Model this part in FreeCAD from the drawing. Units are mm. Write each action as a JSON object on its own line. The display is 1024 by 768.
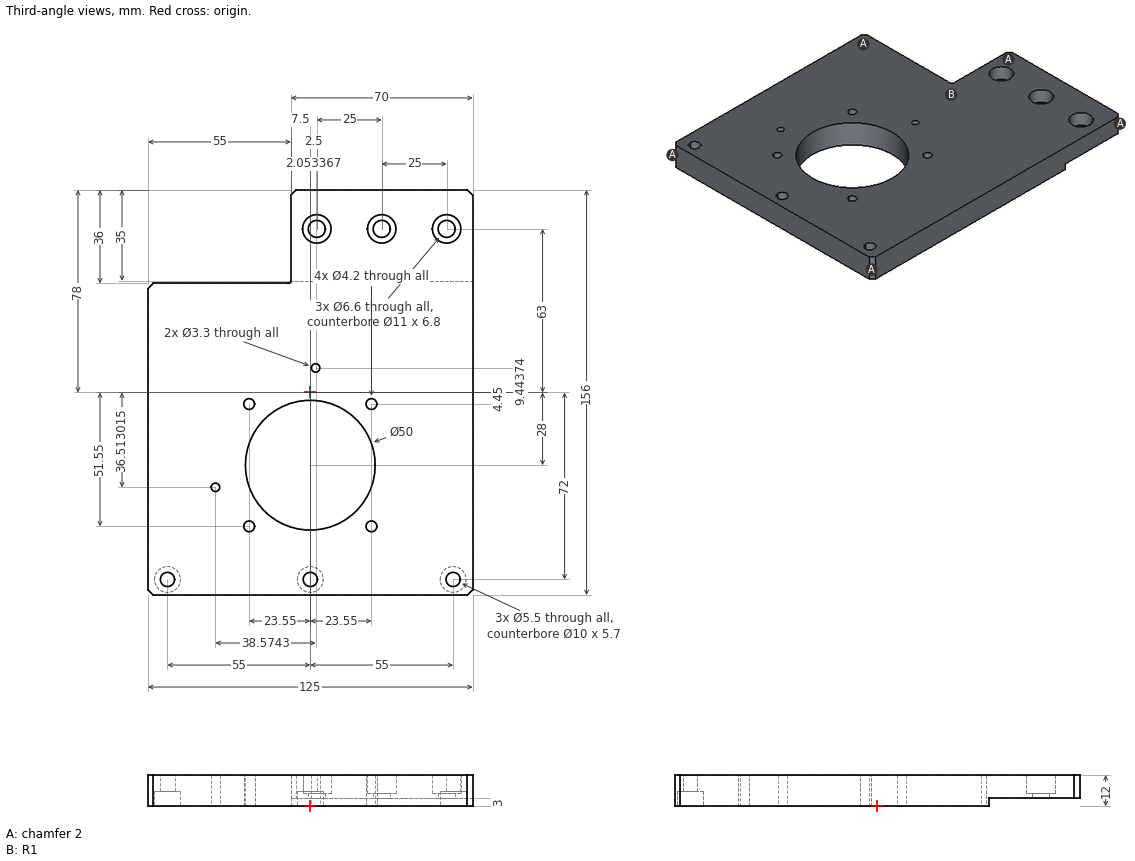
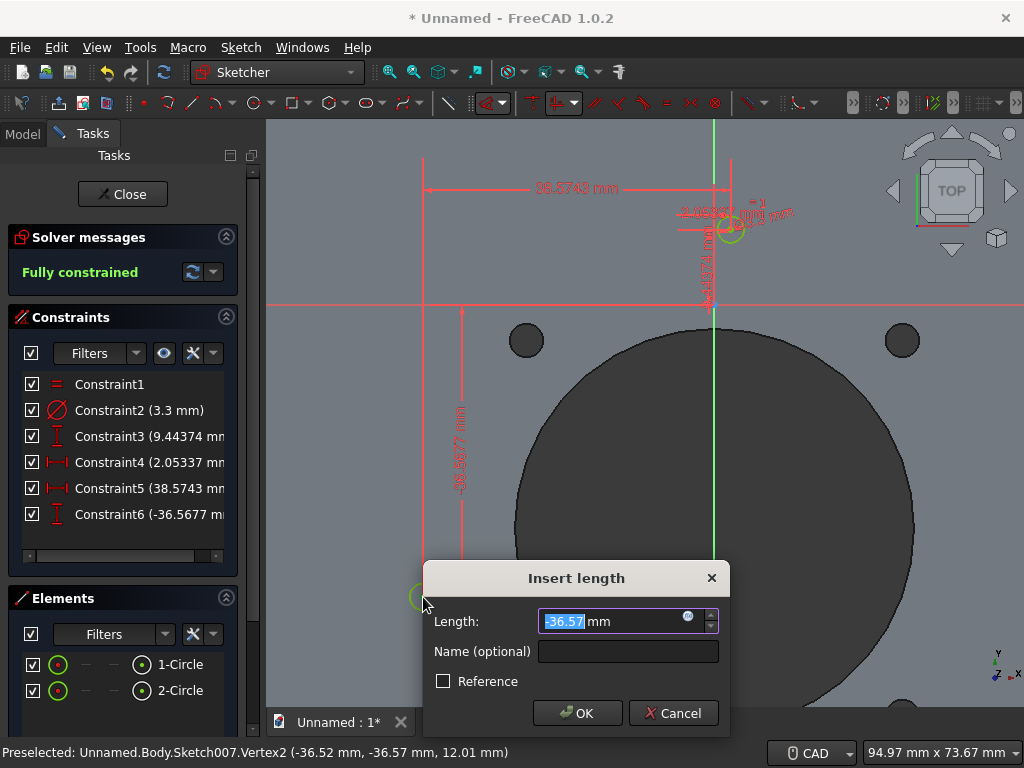
{"action": "type", "text": "-36.513015"}
{"action": "key", "text": "Return"}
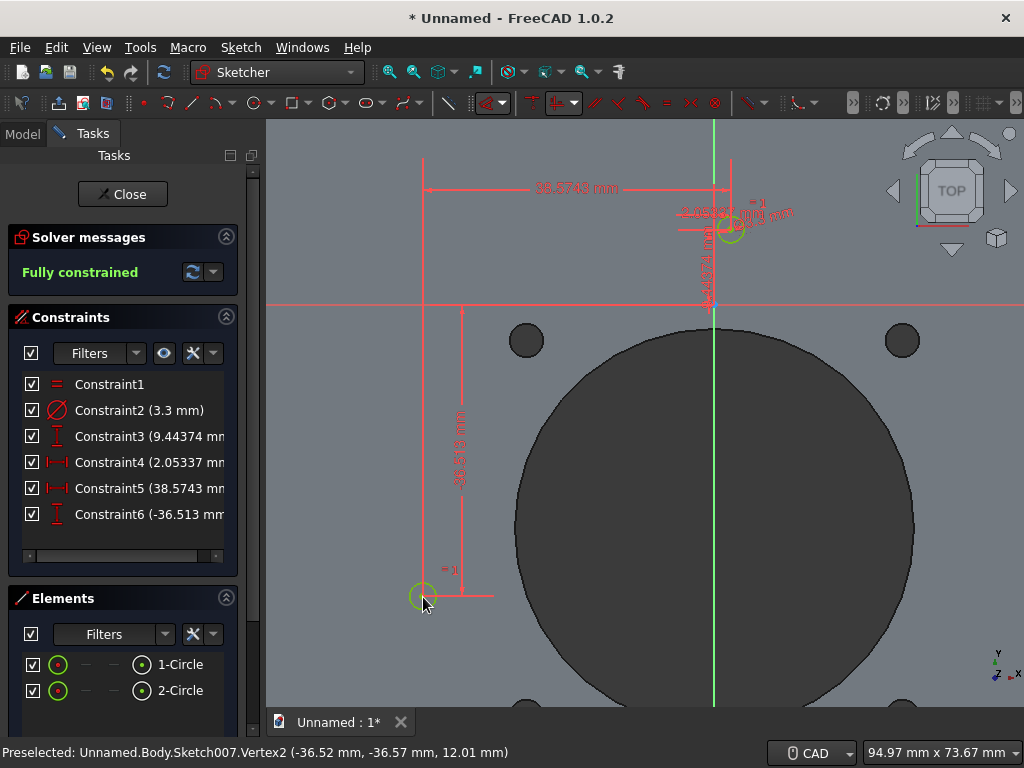
{"action": "left_click", "coordinate": [123, 194]}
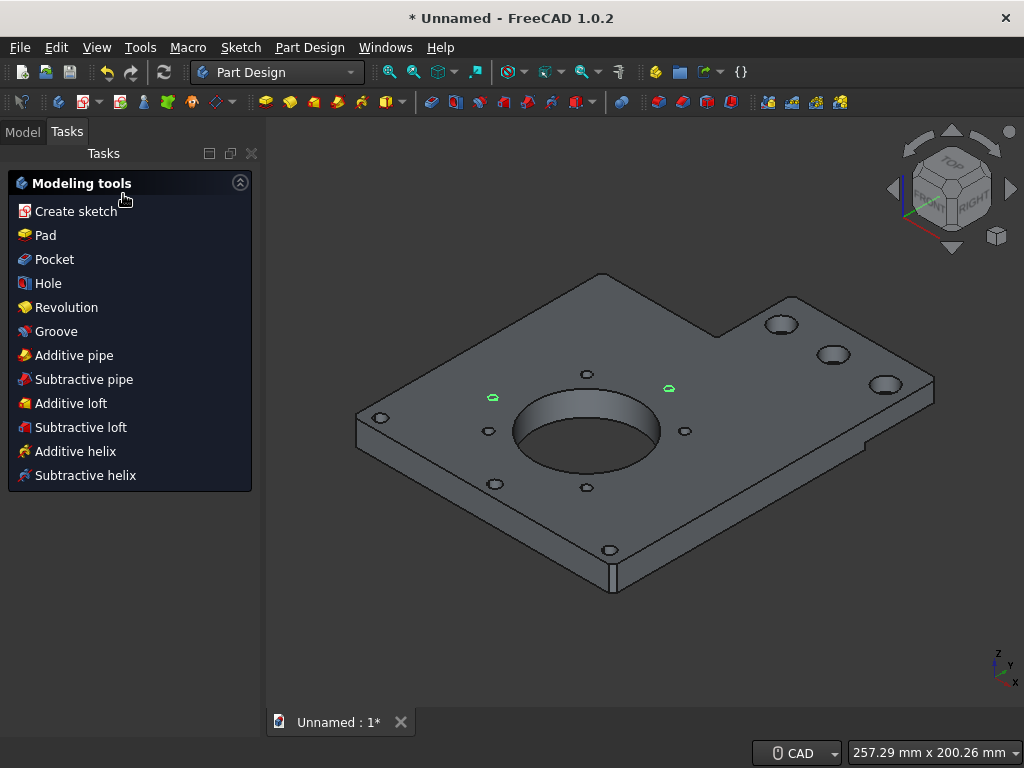
{"action": "left_click", "coordinate": [456, 102]}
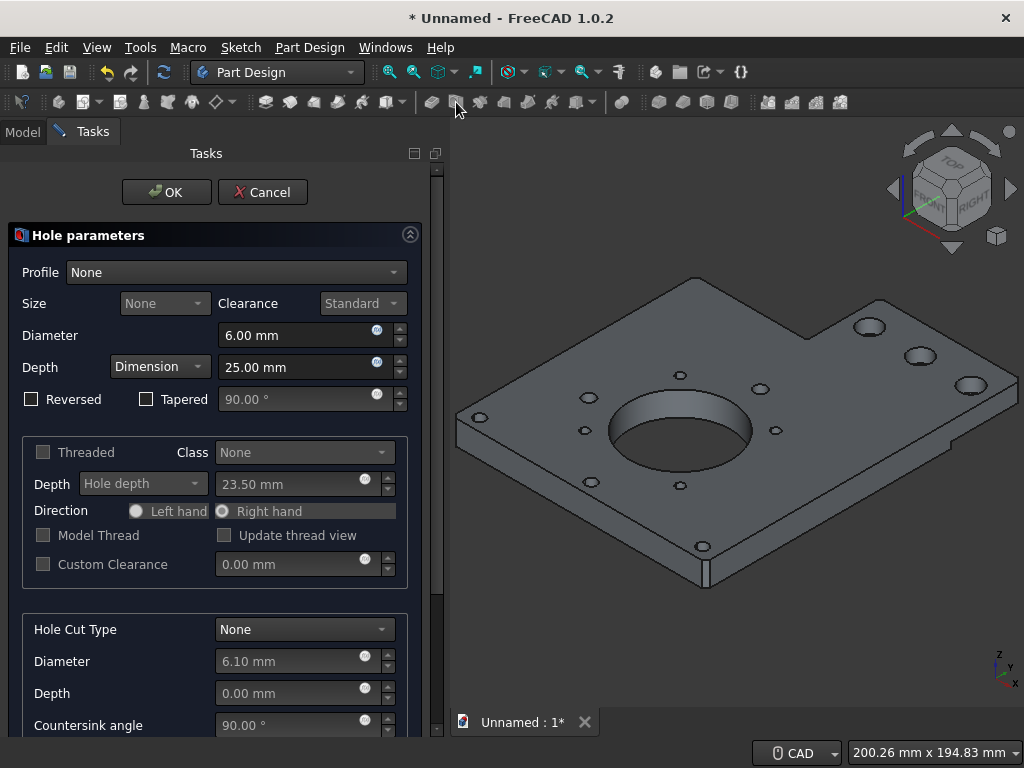
{"action": "triple_click", "coordinate": [305, 335]}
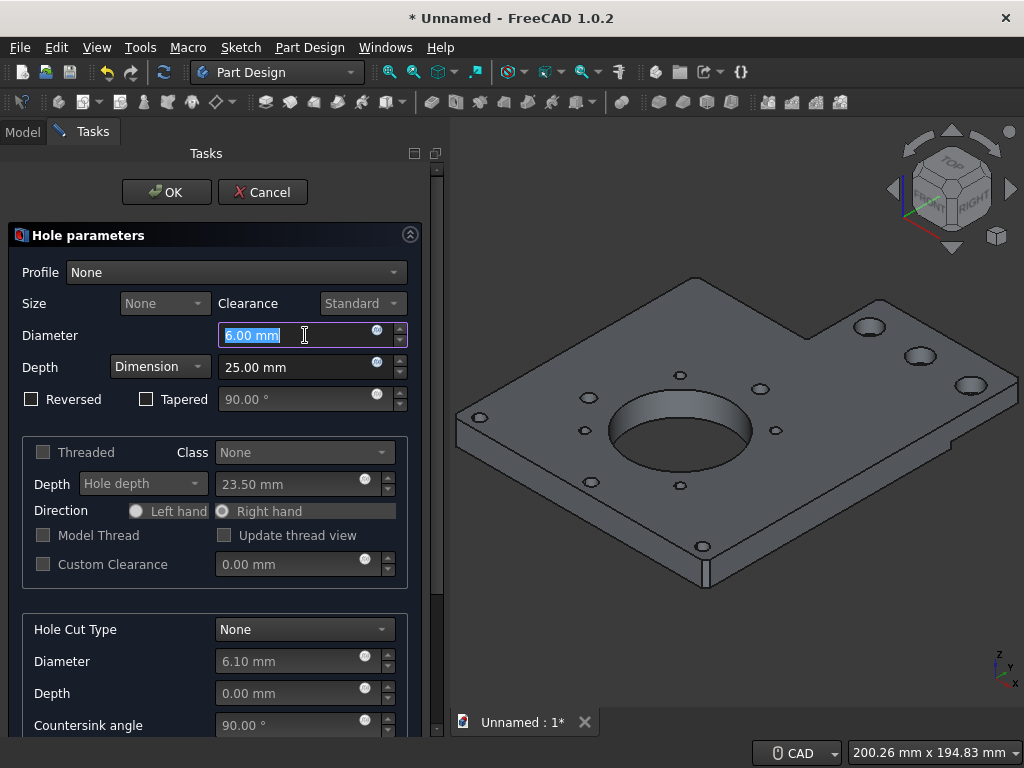
{"action": "type", "text": "3.3"}
{"action": "key", "text": "Tab"}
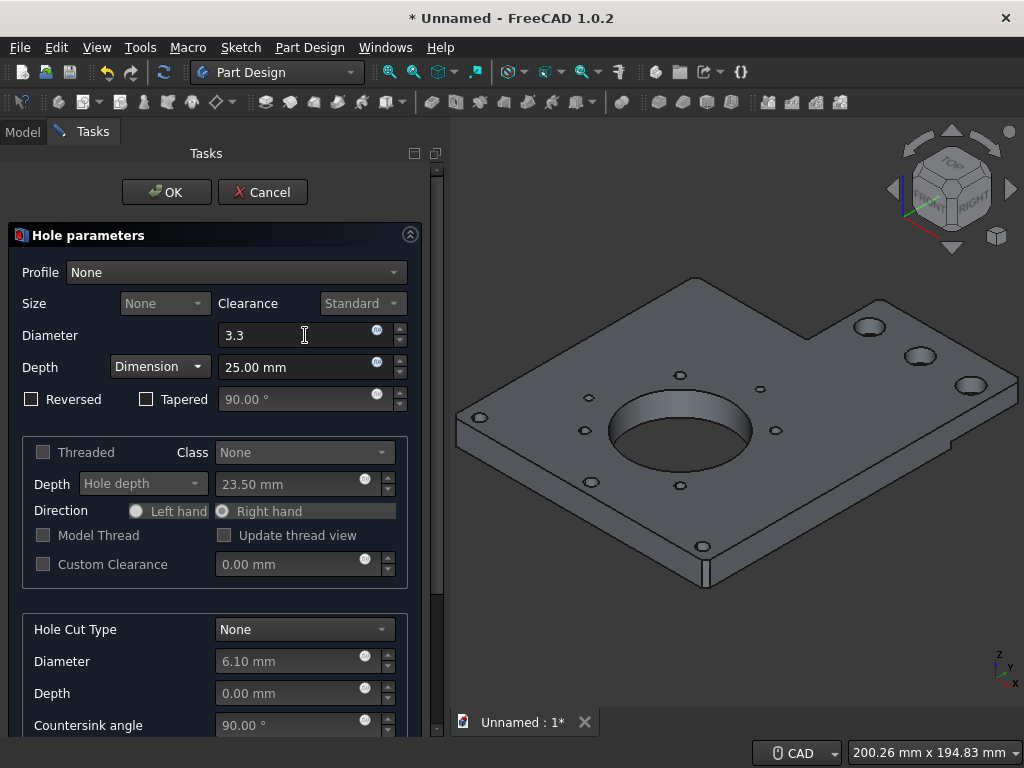
{"action": "left_click", "coordinate": [161, 366]}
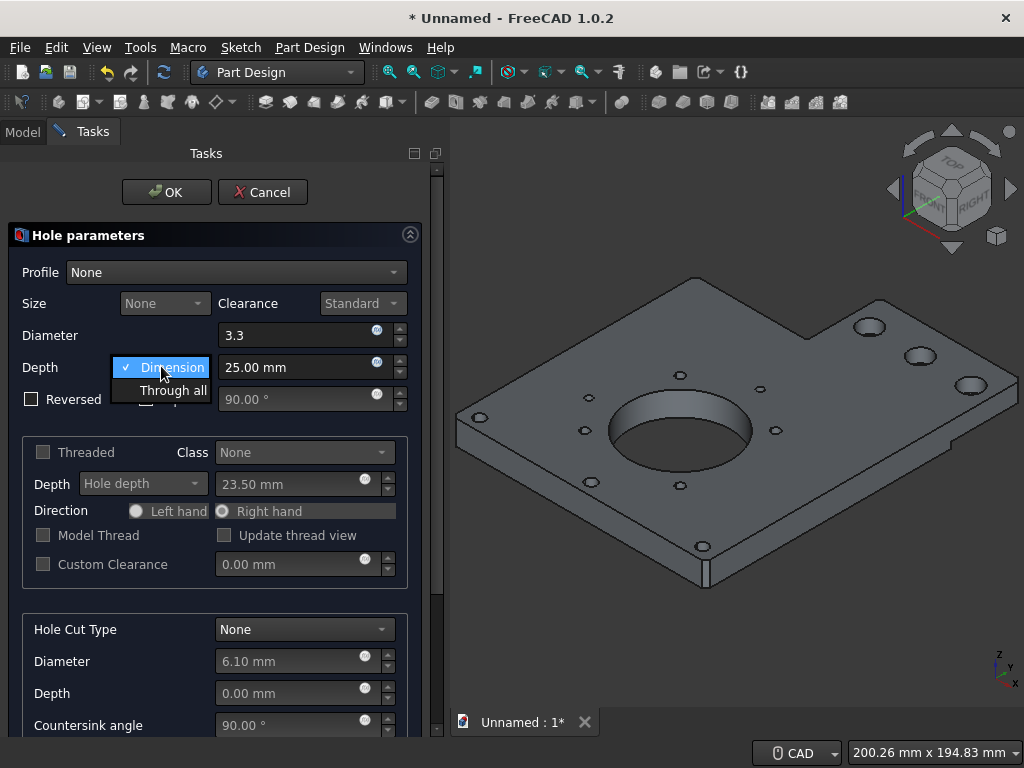
{"action": "left_click", "coordinate": [160, 390]}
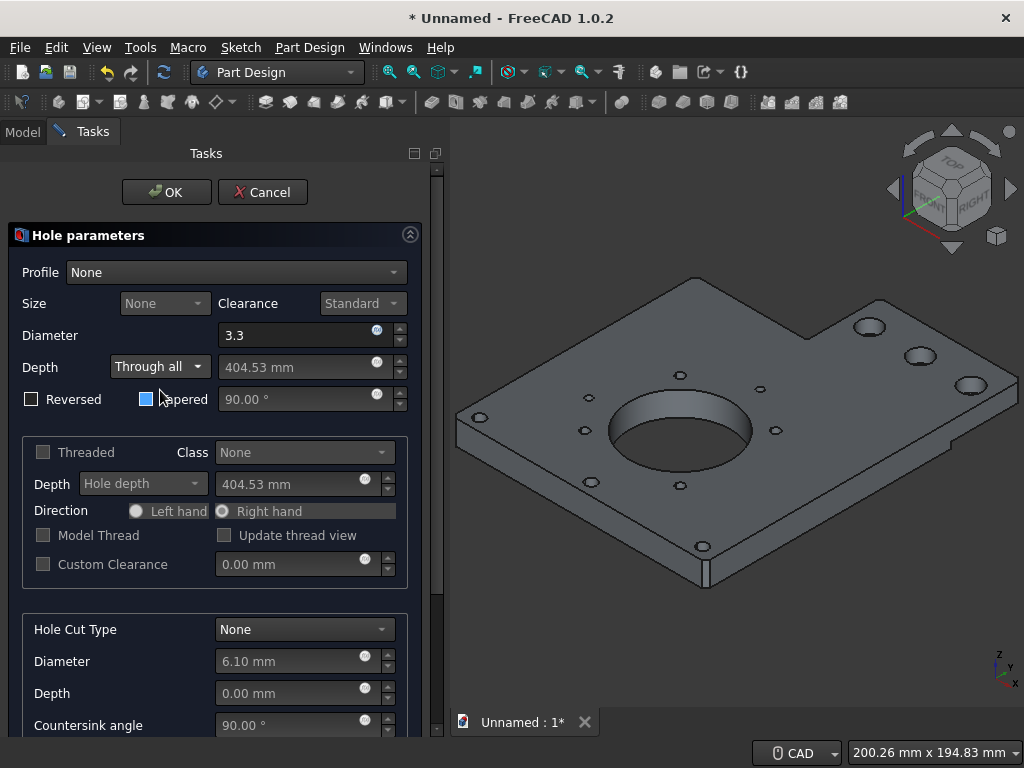
{"action": "left_click", "coordinate": [167, 192]}